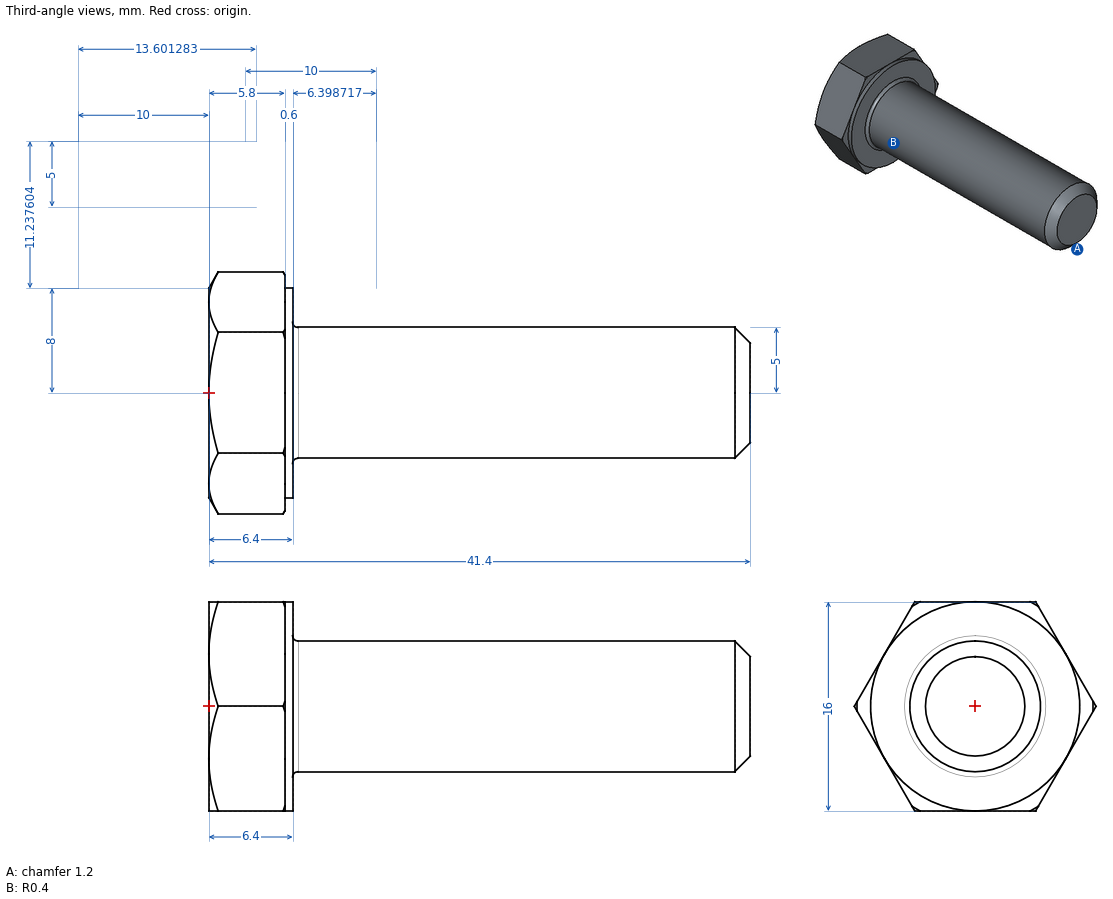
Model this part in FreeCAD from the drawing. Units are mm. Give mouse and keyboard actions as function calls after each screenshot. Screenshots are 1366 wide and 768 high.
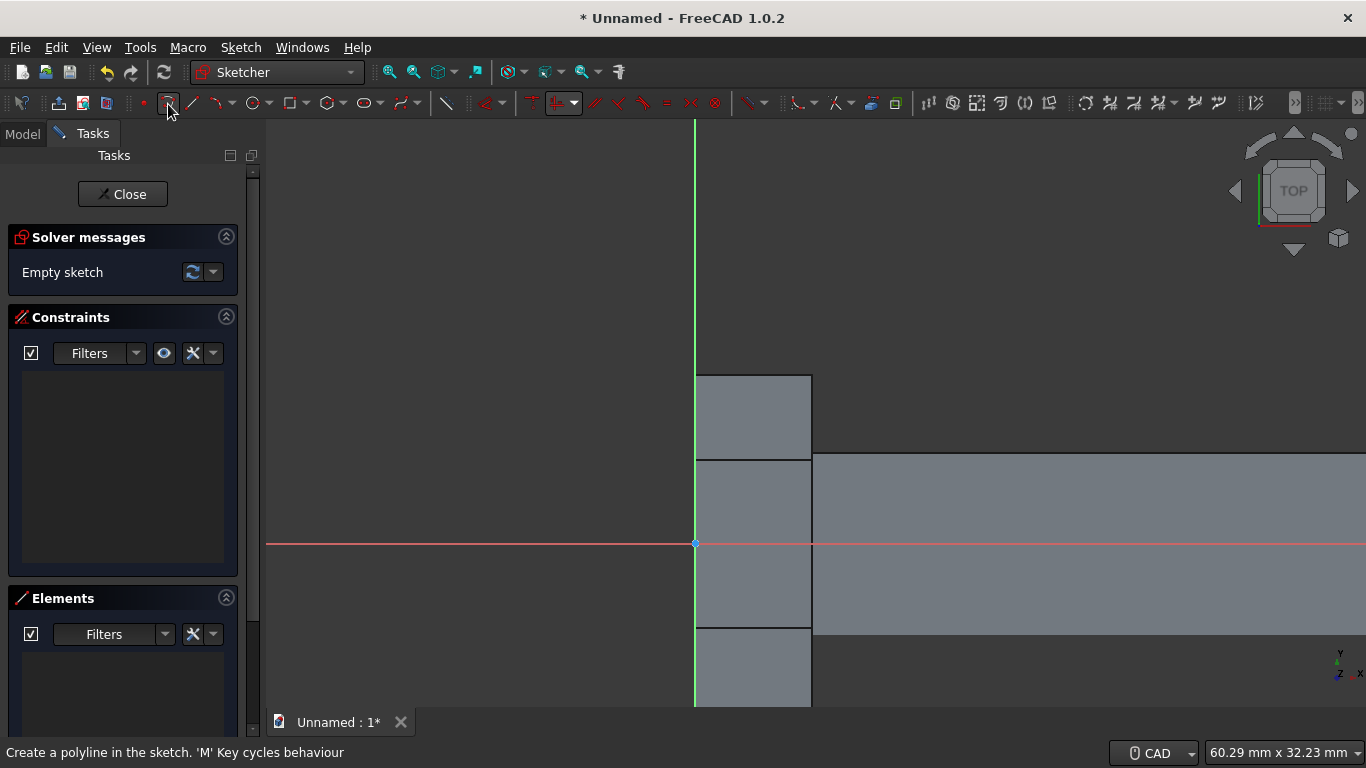
click(695, 398)
click(761, 284)
click(761, 193)
click(513, 193)
click(513, 398)
click(695, 399)
key(Escape)
key(Escape)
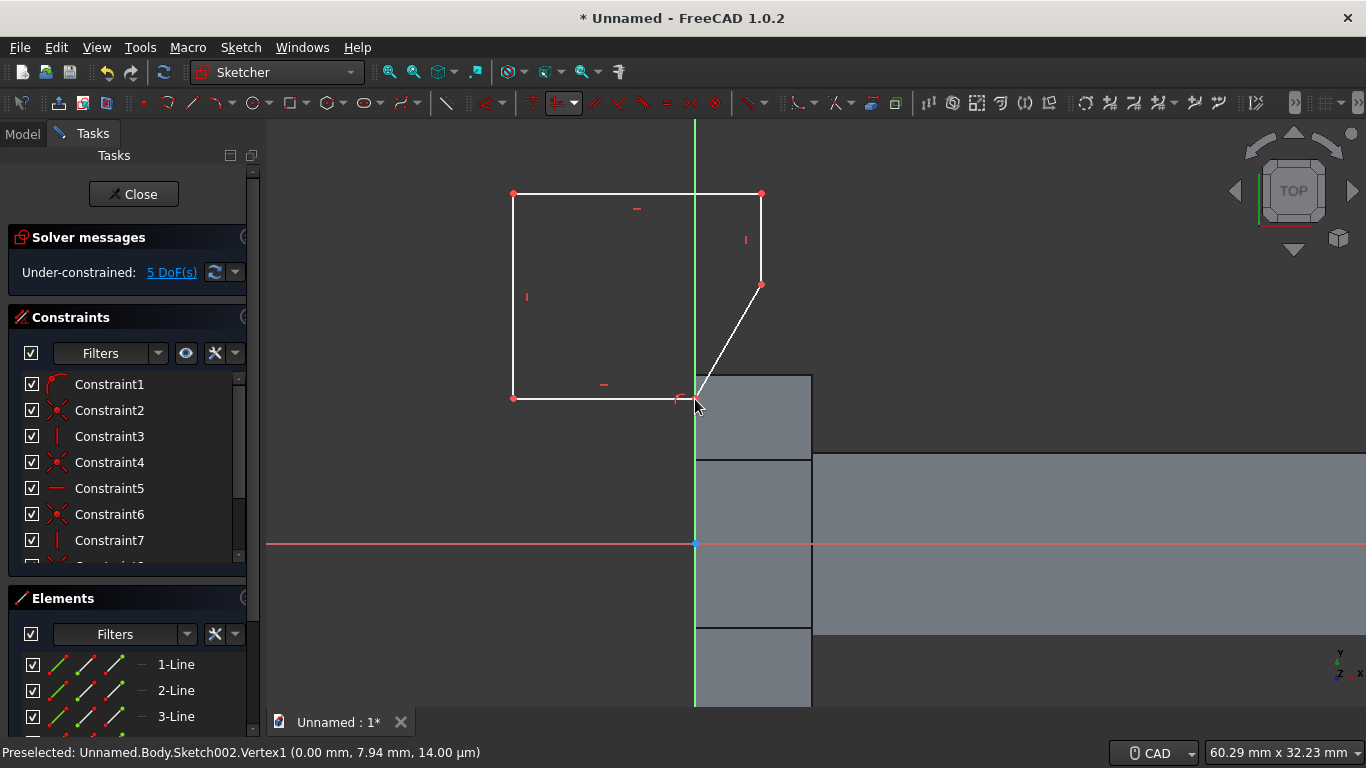
click(486, 104)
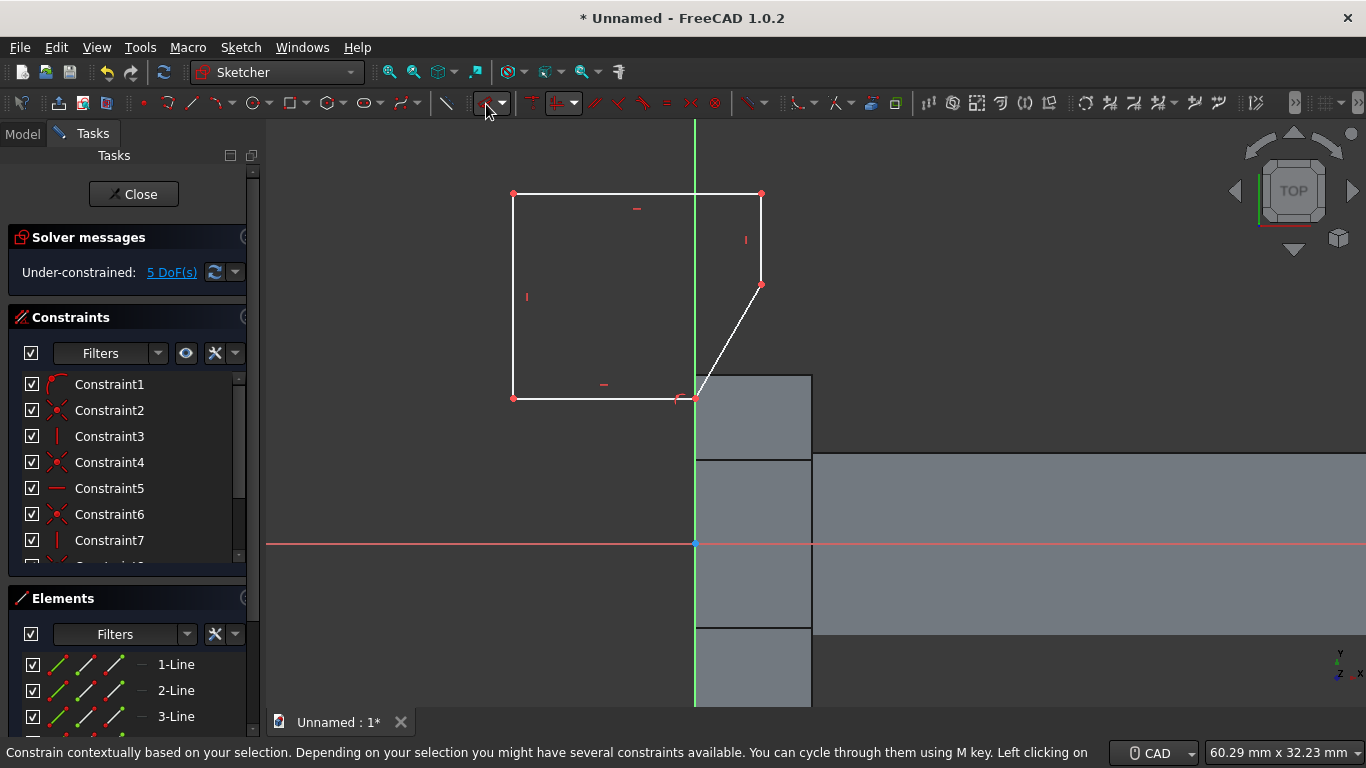
click(761, 258)
click(795, 240)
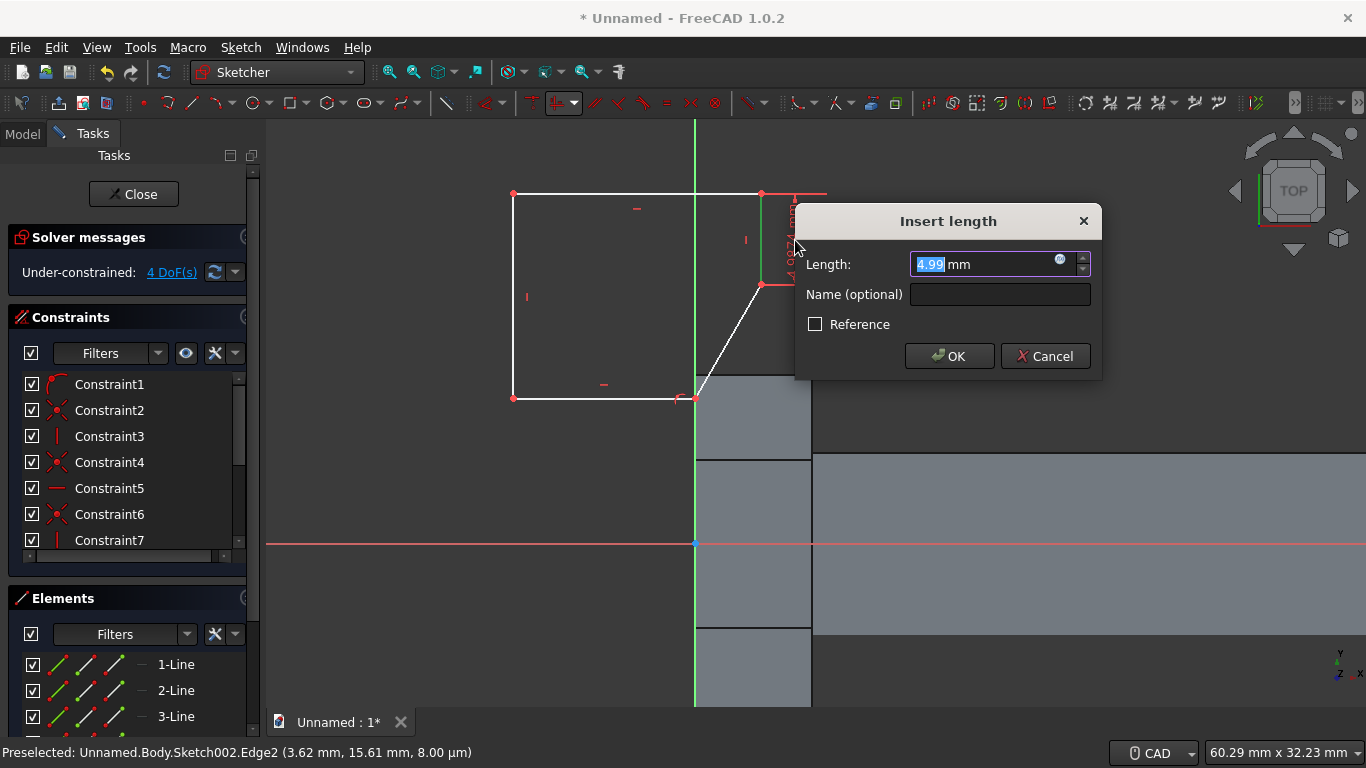
text(5)
key(Return)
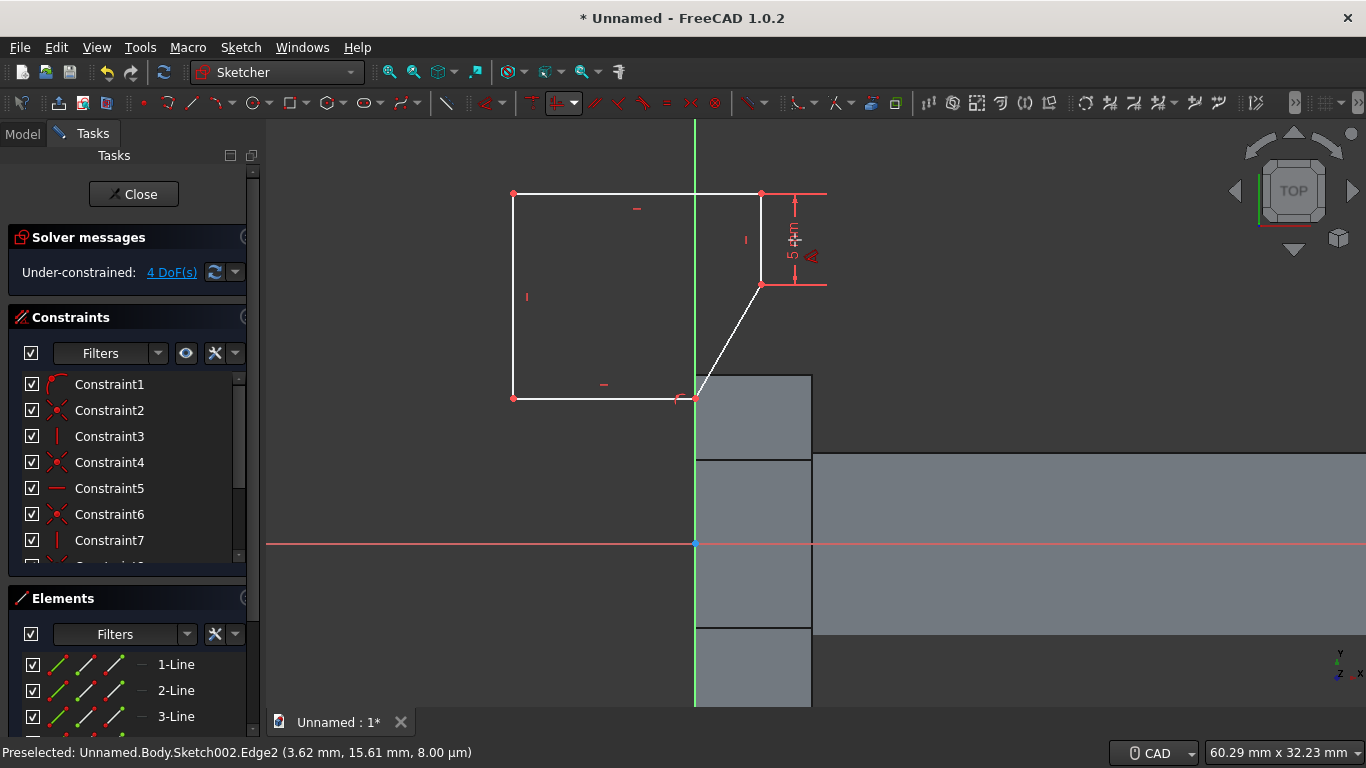
click(568, 399)
click(604, 433)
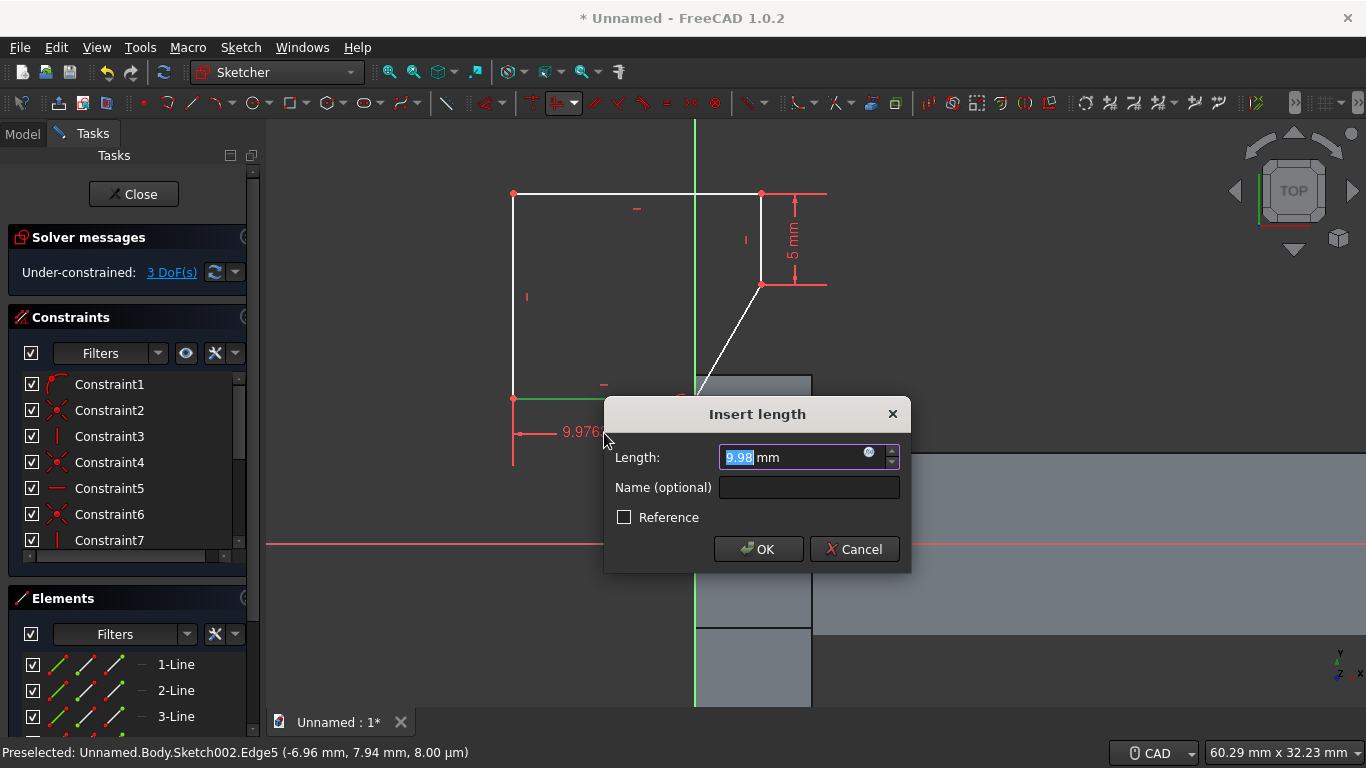
text(10)
key(Return)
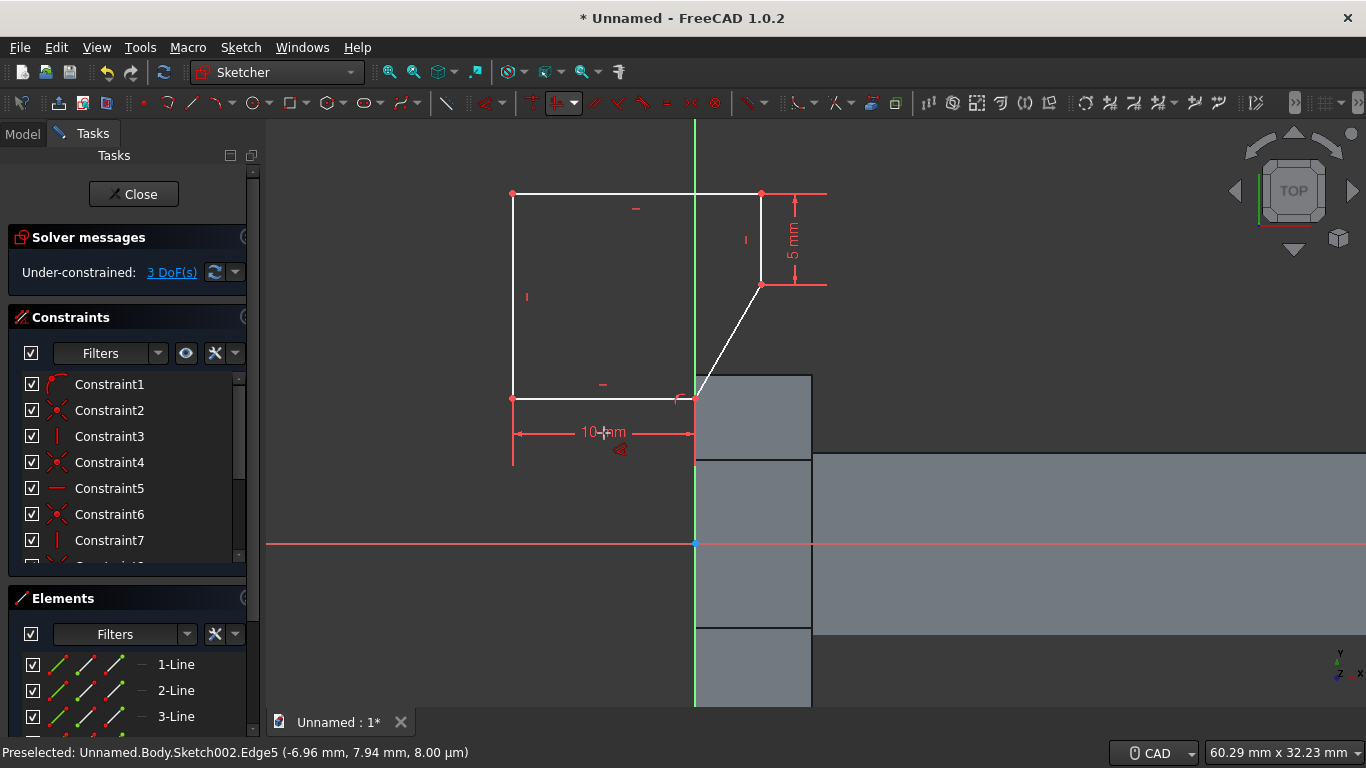
click(695, 399)
click(729, 471)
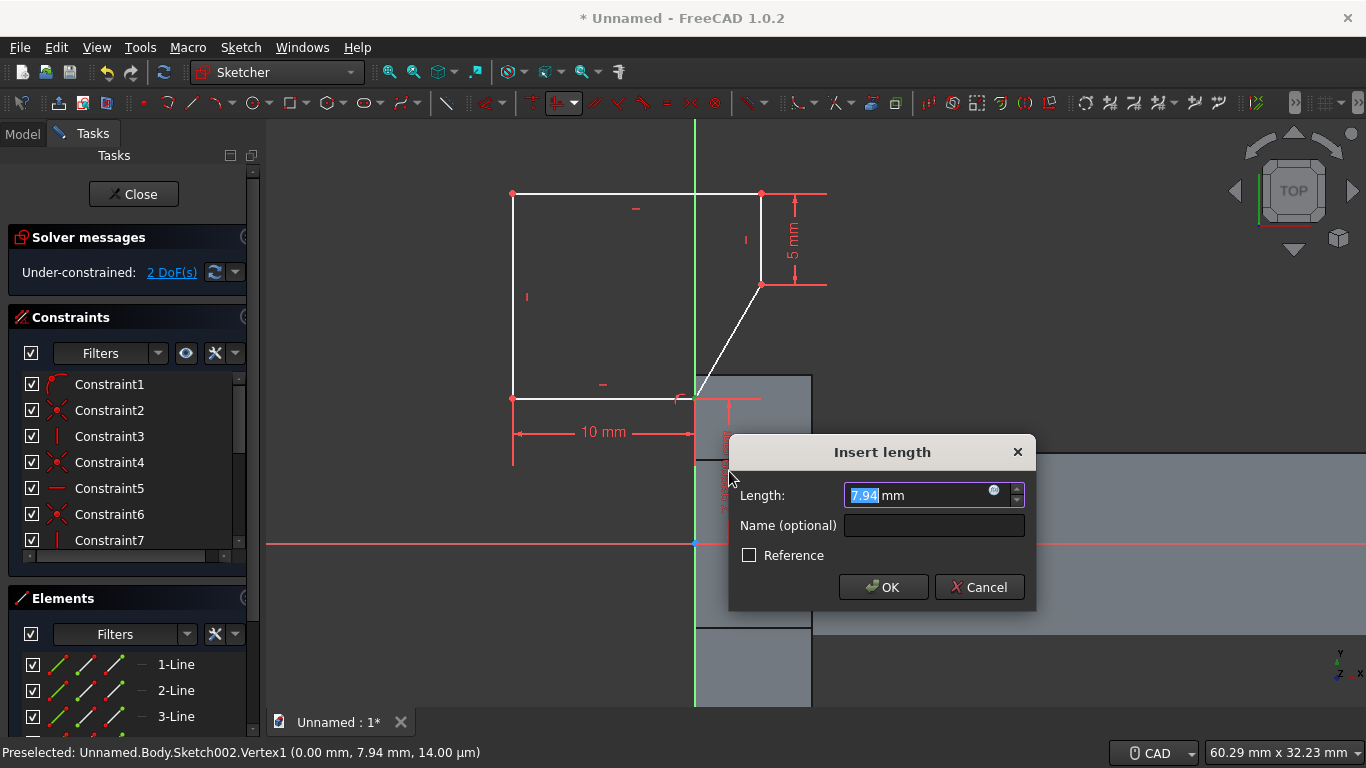
text(8)
key(Return)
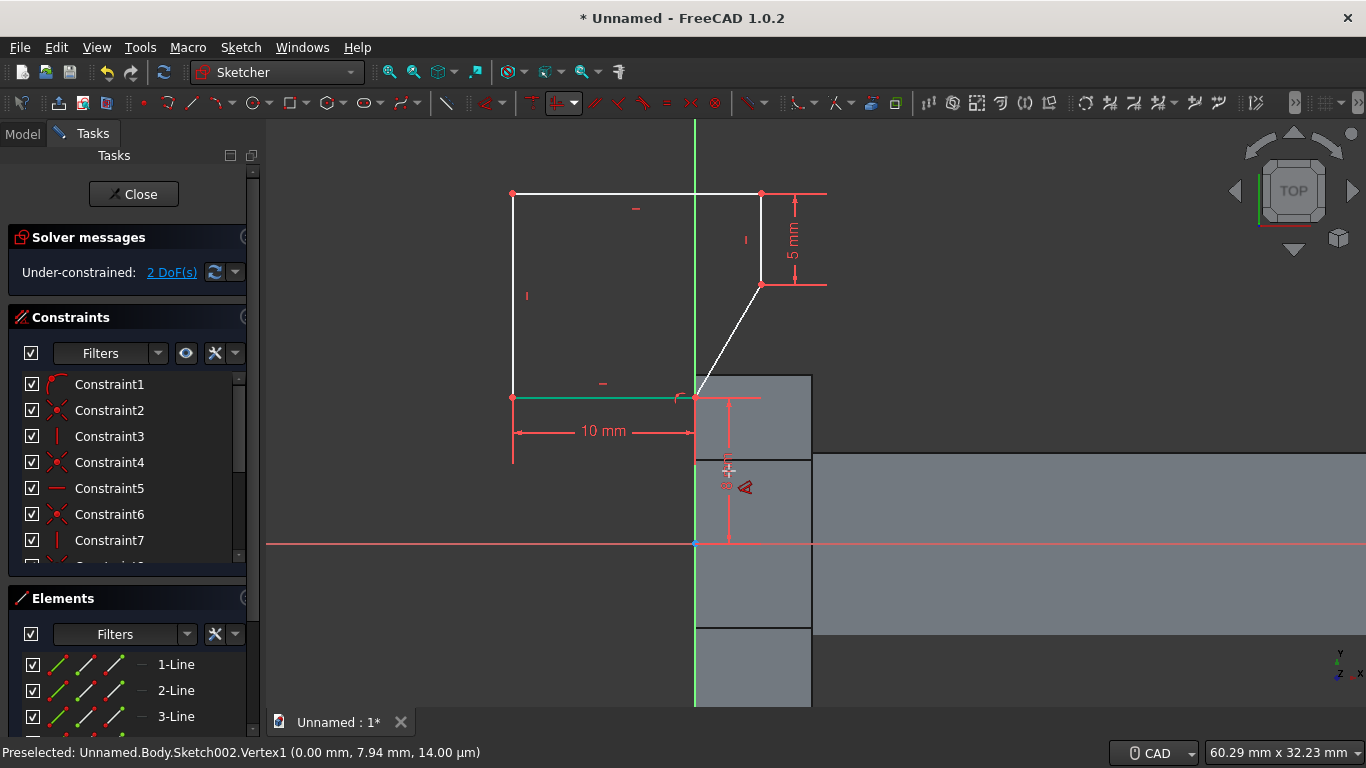
click(587, 194)
click(637, 160)